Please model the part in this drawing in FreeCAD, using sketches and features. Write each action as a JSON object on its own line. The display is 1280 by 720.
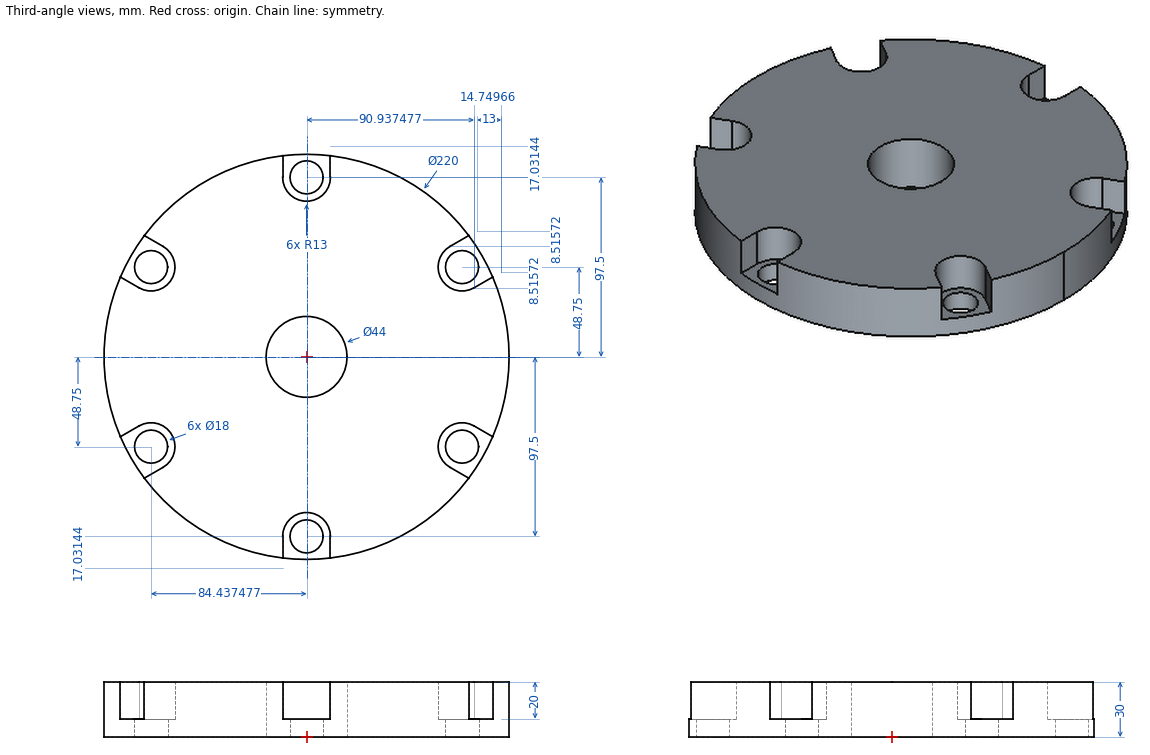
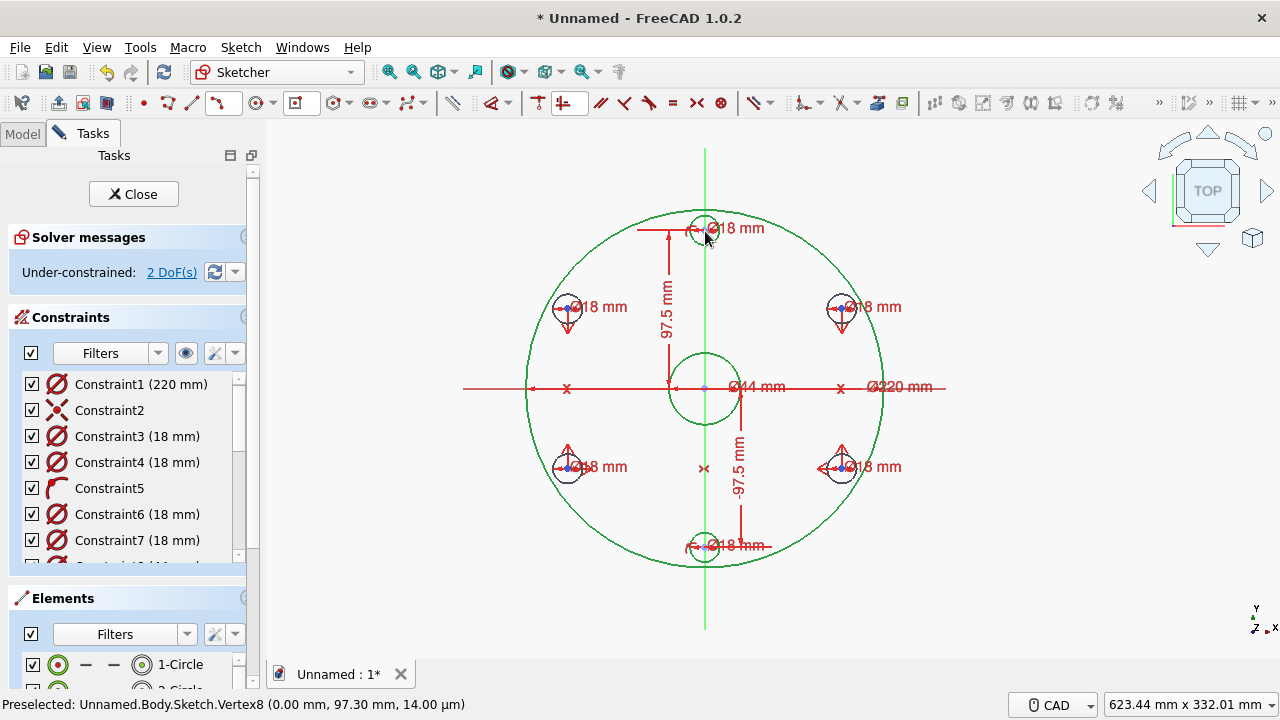
{"action": "left_click", "coordinate": [568, 469]}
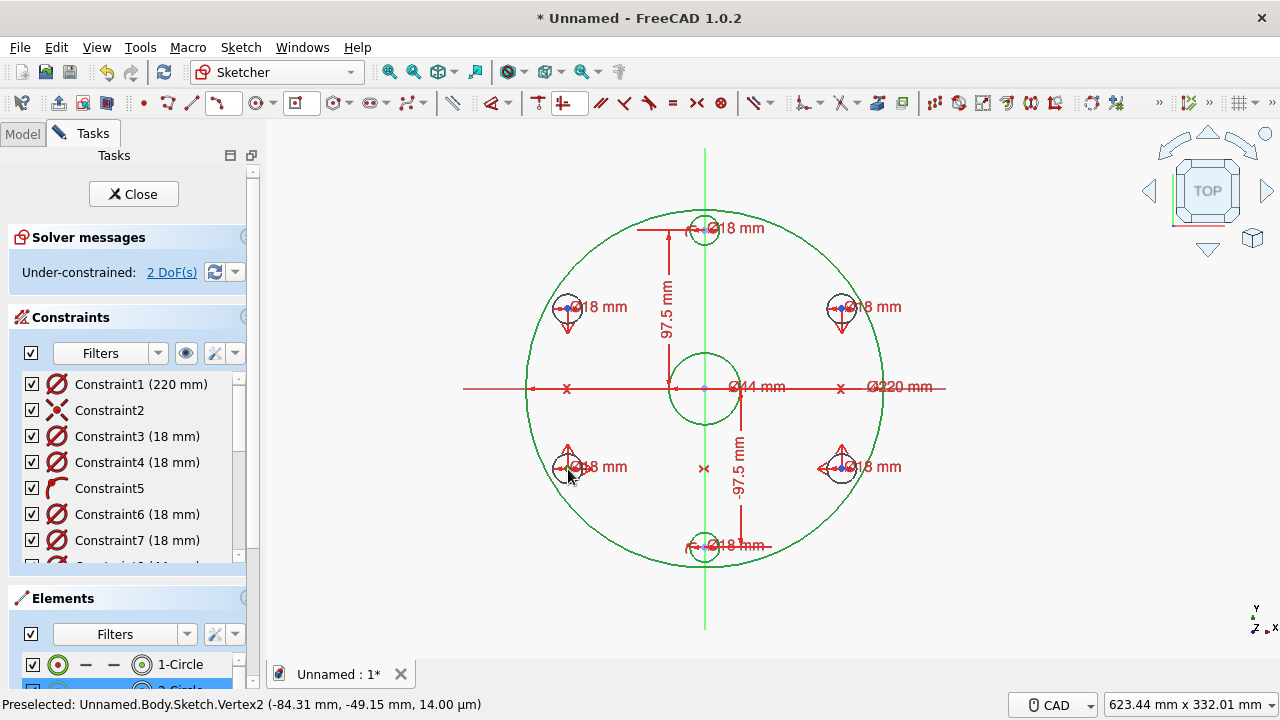
{"action": "key", "text": "i"}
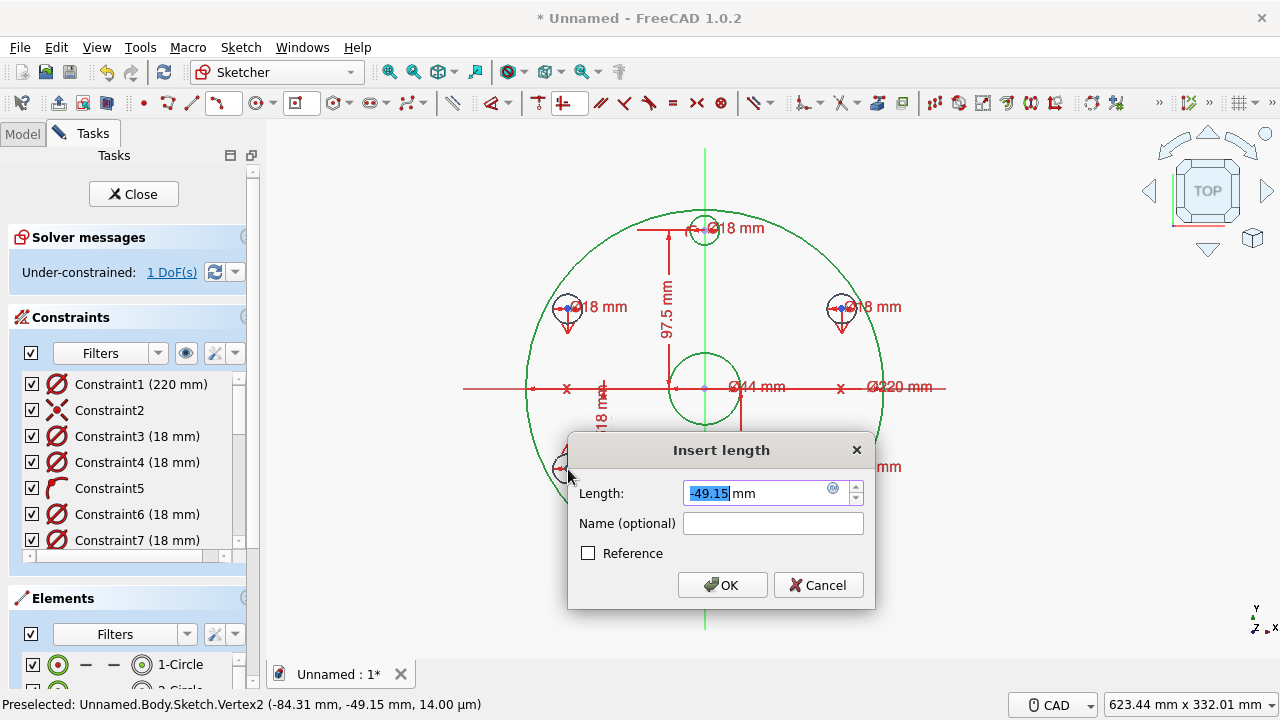
{"action": "type", "text": "-48.75"}
{"action": "key", "text": "Return"}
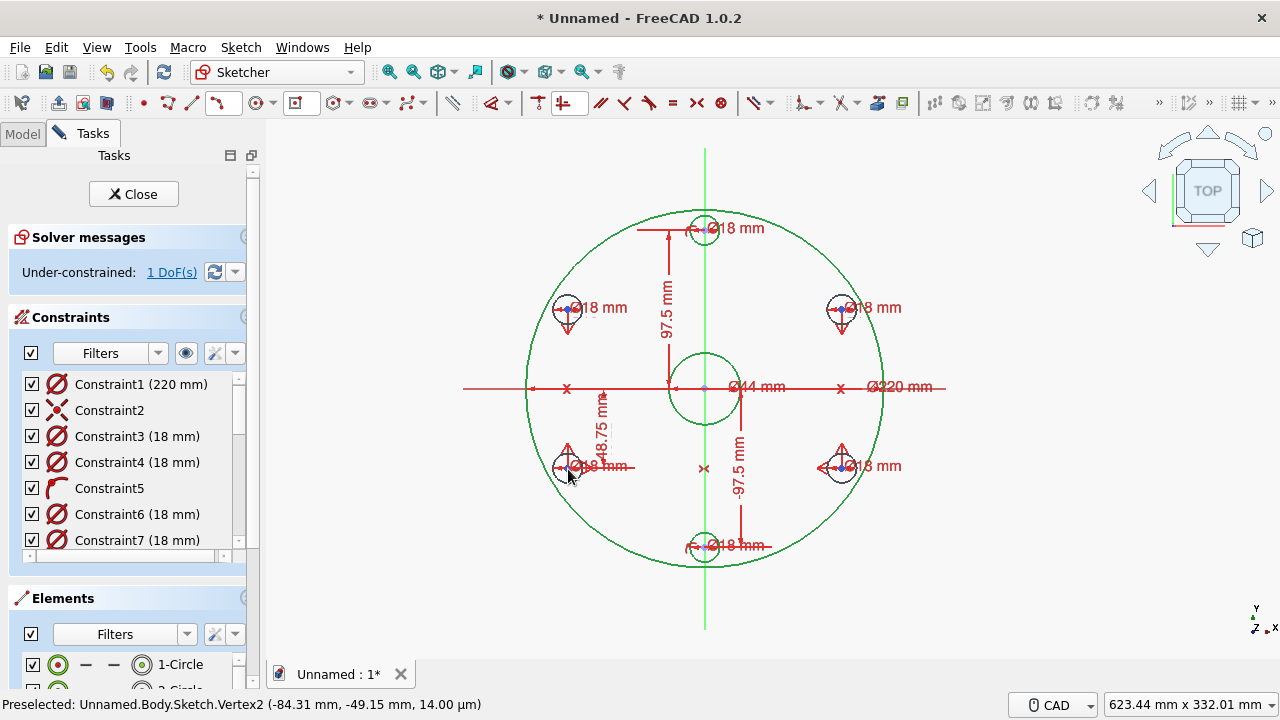
{"action": "left_click", "coordinate": [568, 468]}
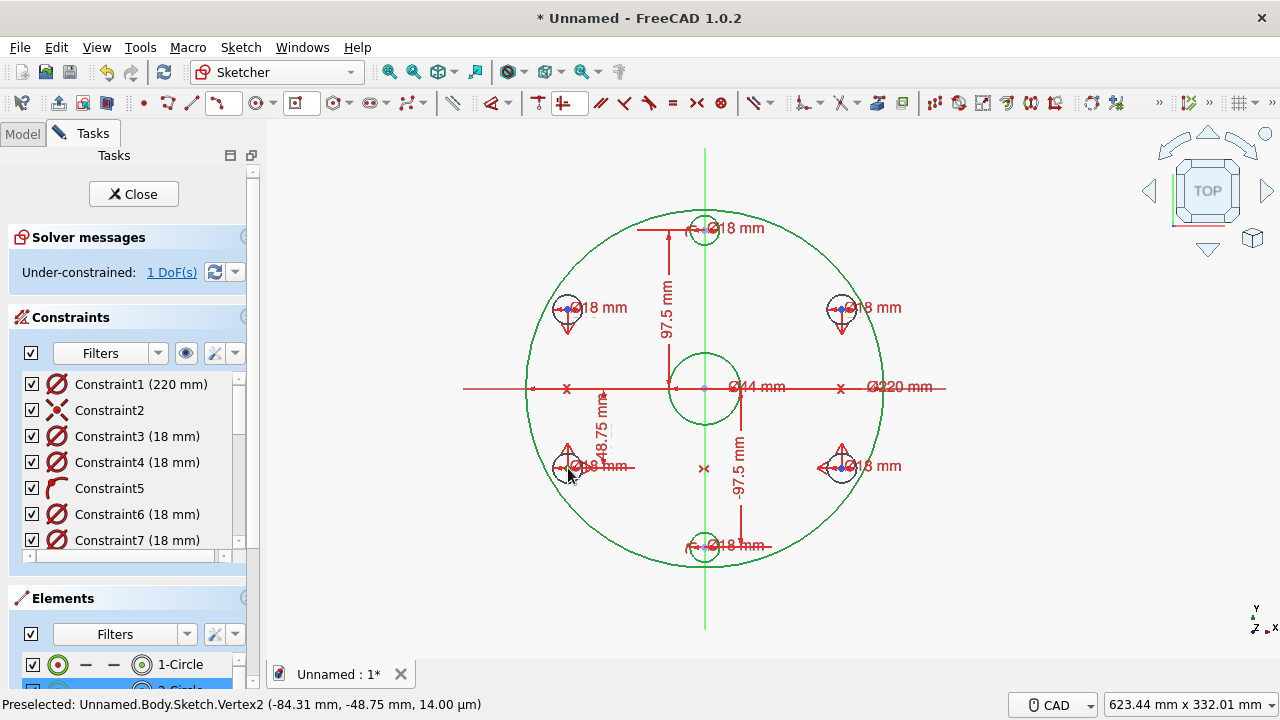
{"action": "left_click", "coordinate": [510, 104]}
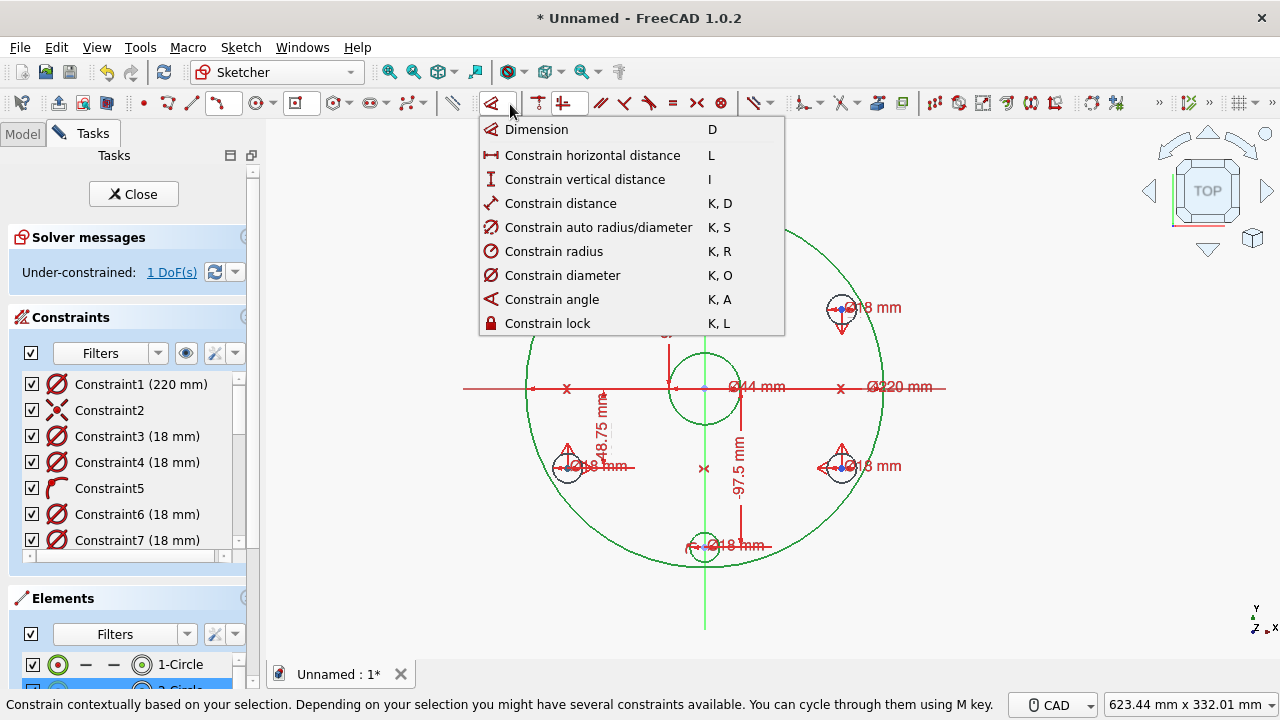
{"action": "left_click", "coordinate": [632, 155]}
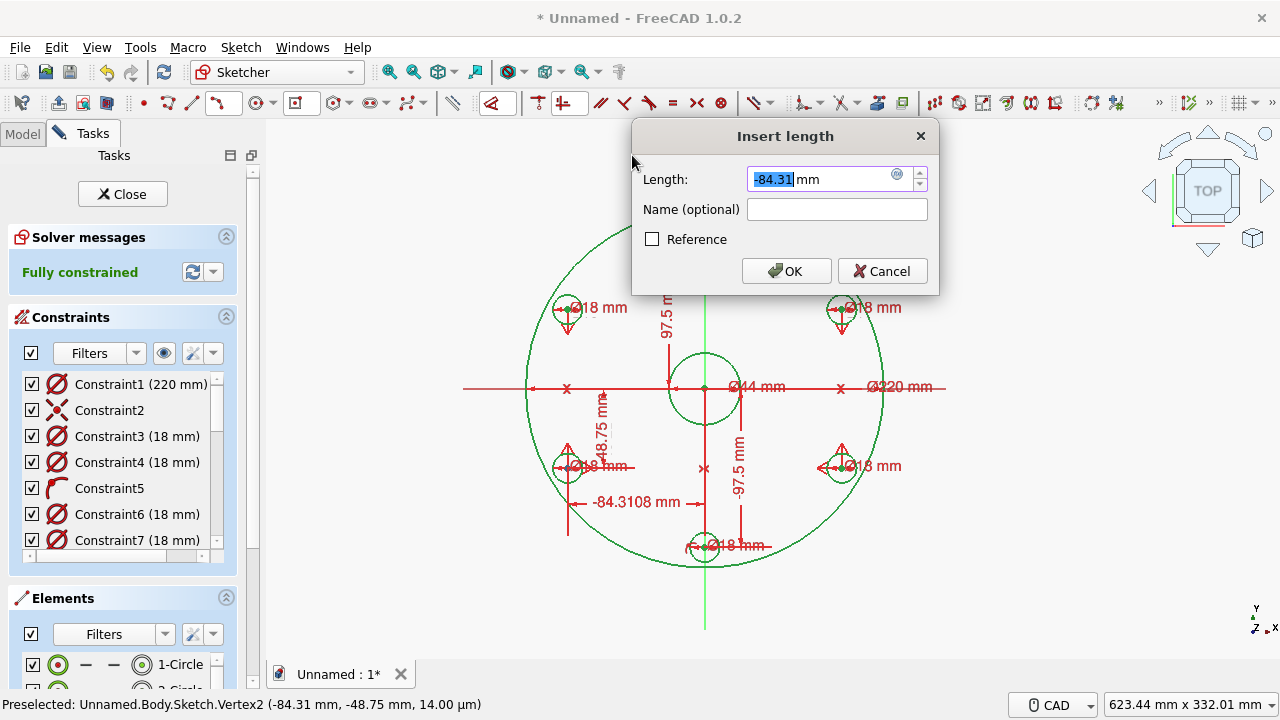
{"action": "type", "text": "-84.437477"}
{"action": "key", "text": "Return"}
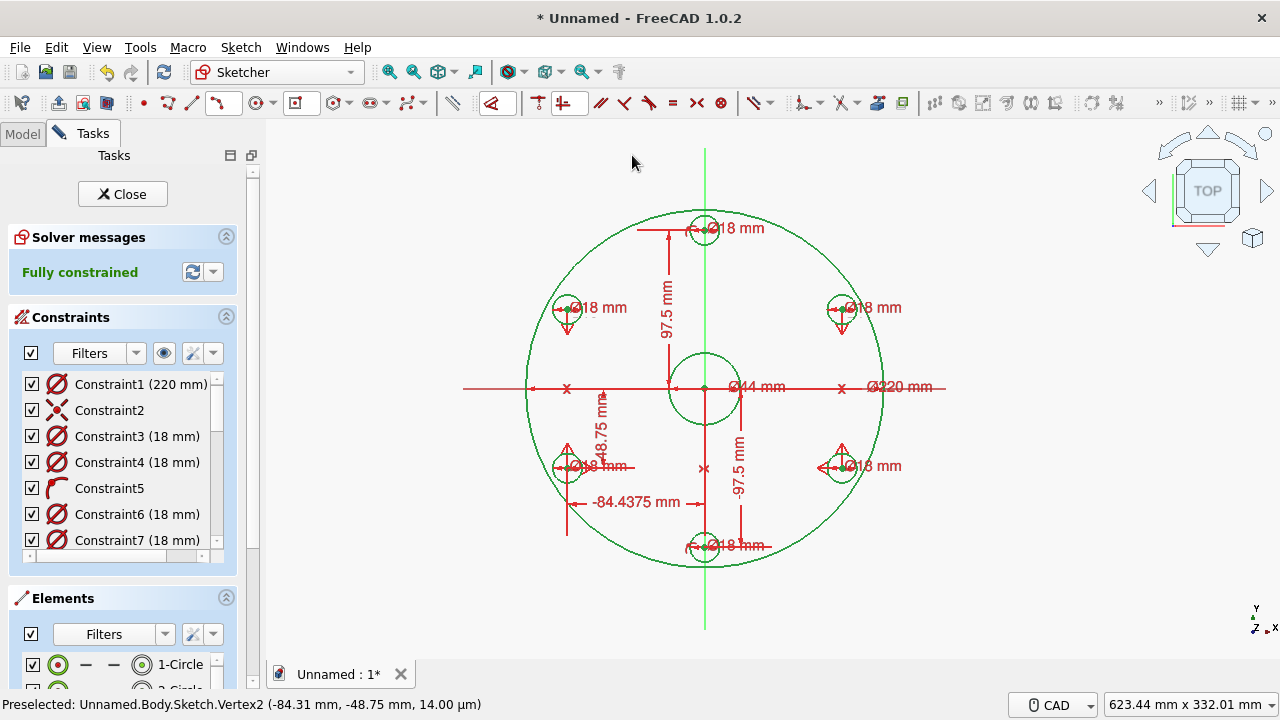
{"action": "left_click", "coordinate": [123, 194]}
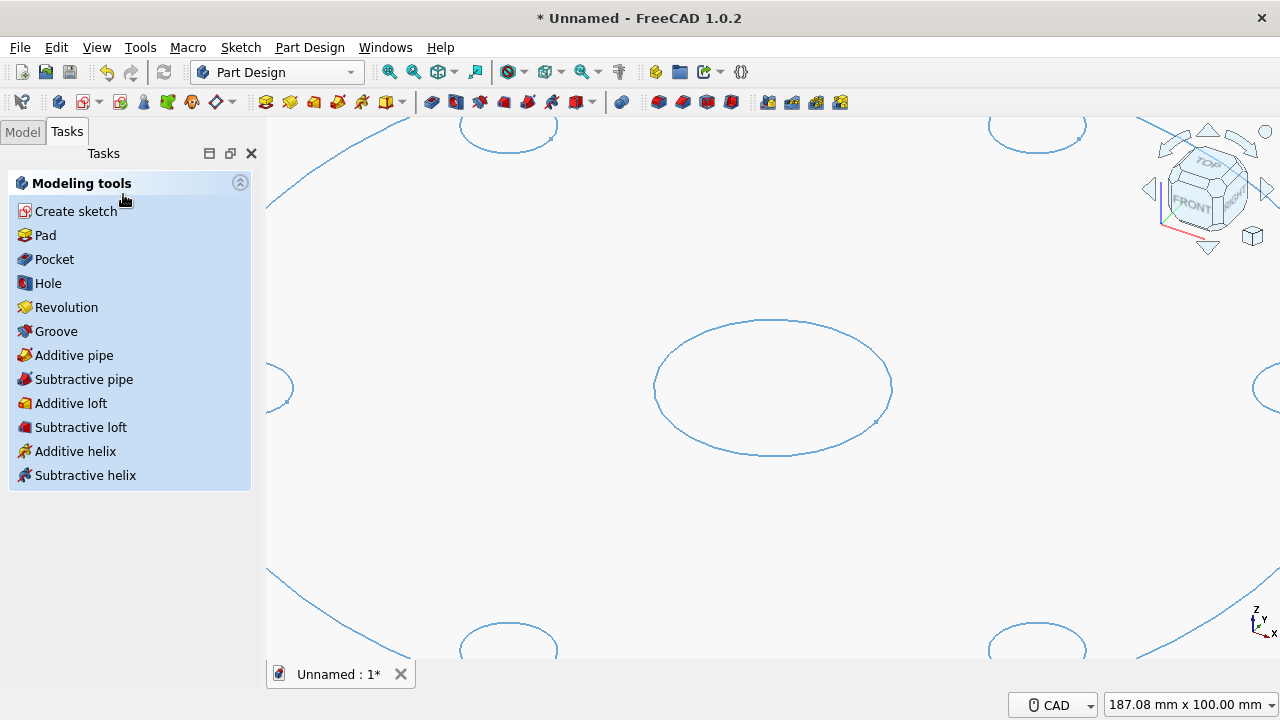
{"action": "left_click", "coordinate": [266, 102]}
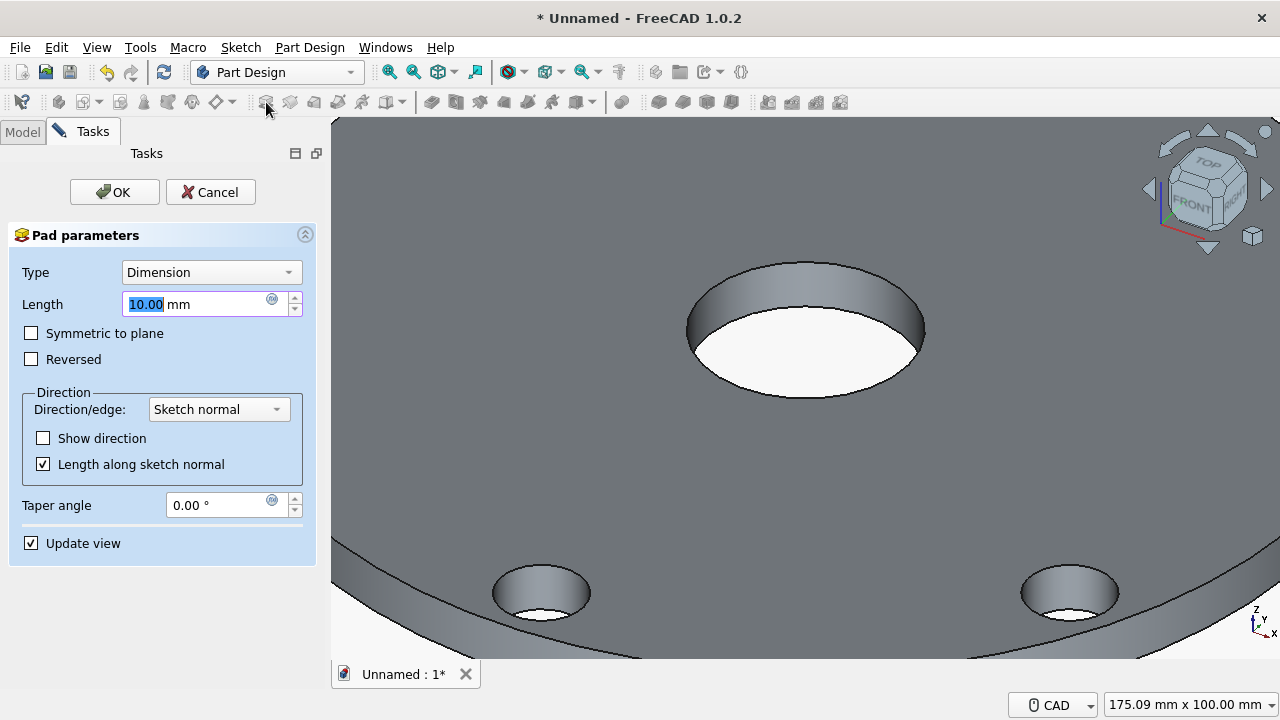
{"action": "type", "text": "30"}
{"action": "key", "text": "Tab"}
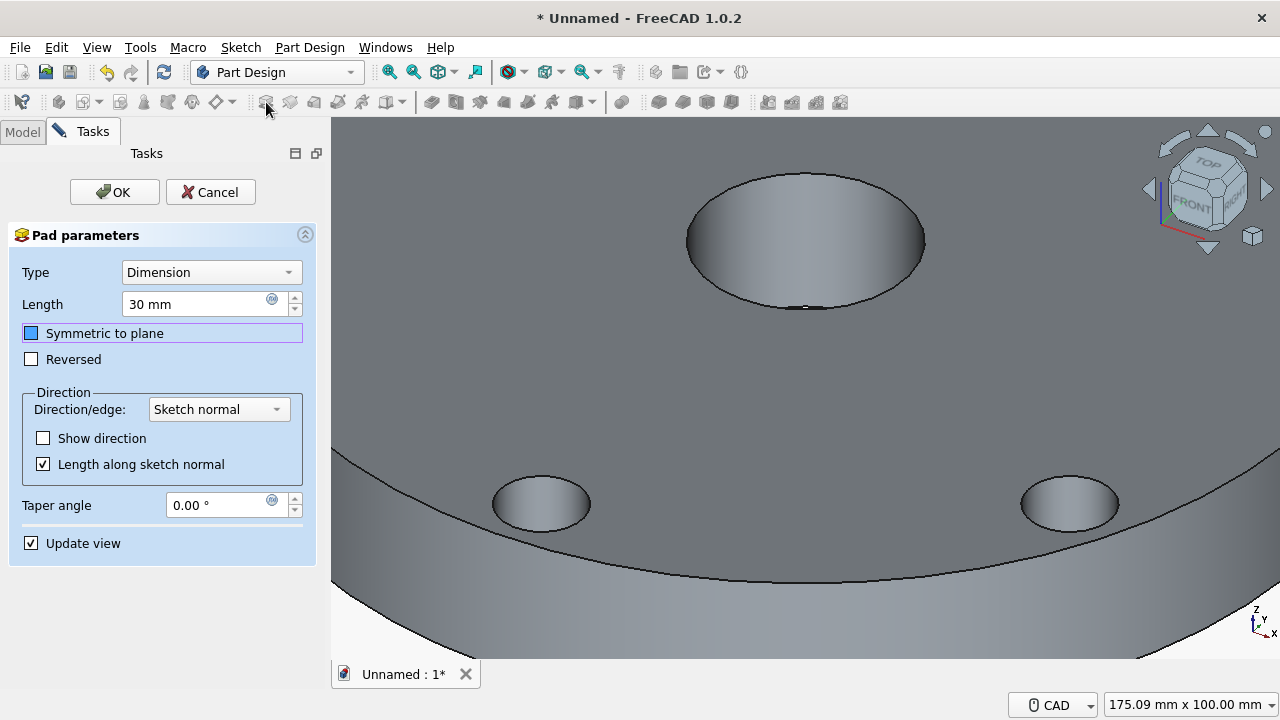
{"action": "left_click", "coordinate": [115, 192]}